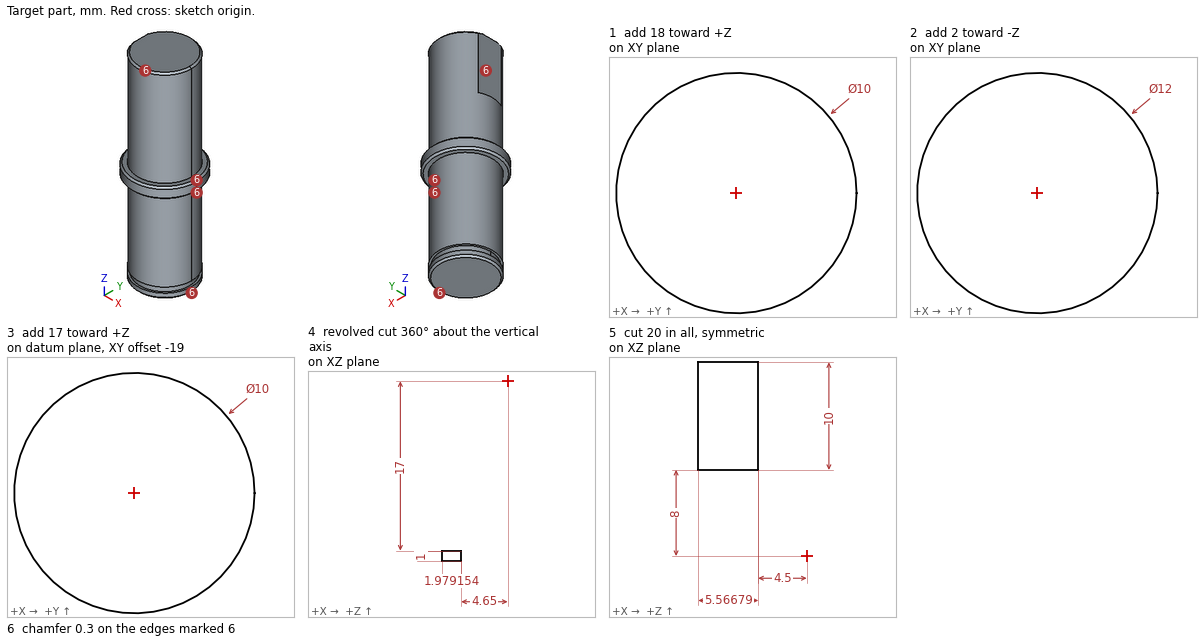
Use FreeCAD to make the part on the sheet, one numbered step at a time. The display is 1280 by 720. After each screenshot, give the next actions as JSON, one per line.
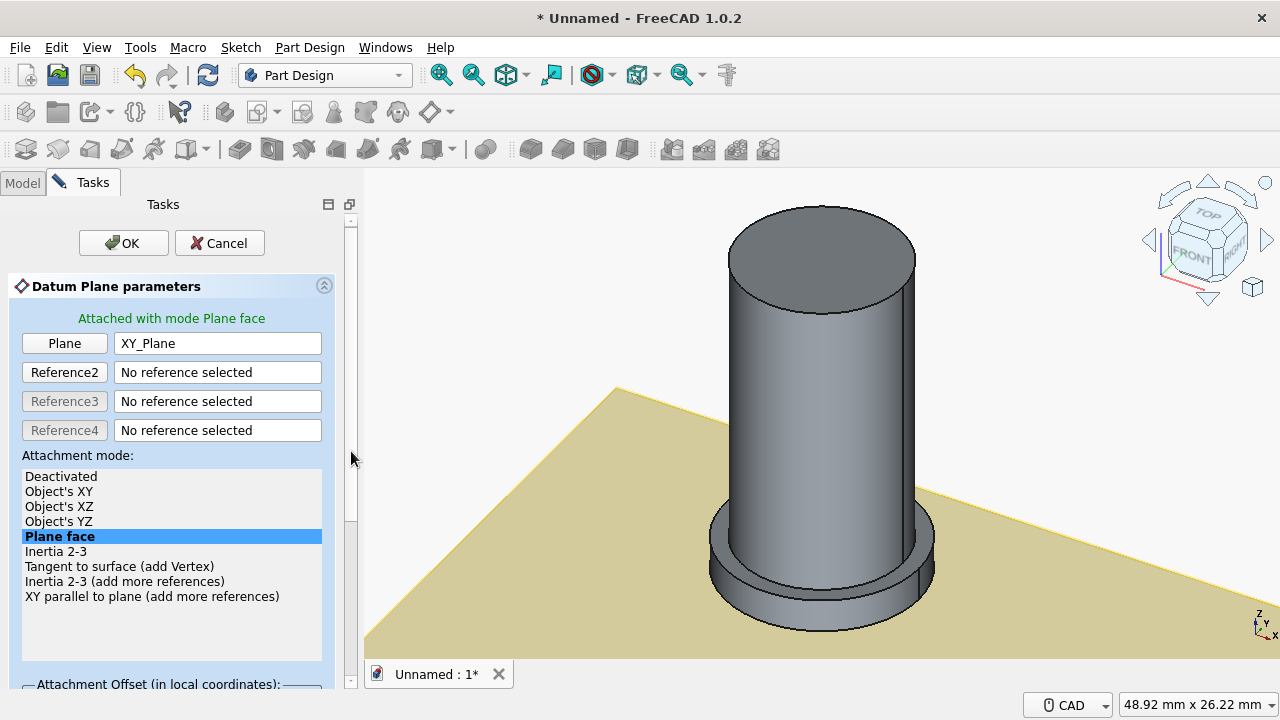
{"action": "left_click", "coordinate": [124, 243]}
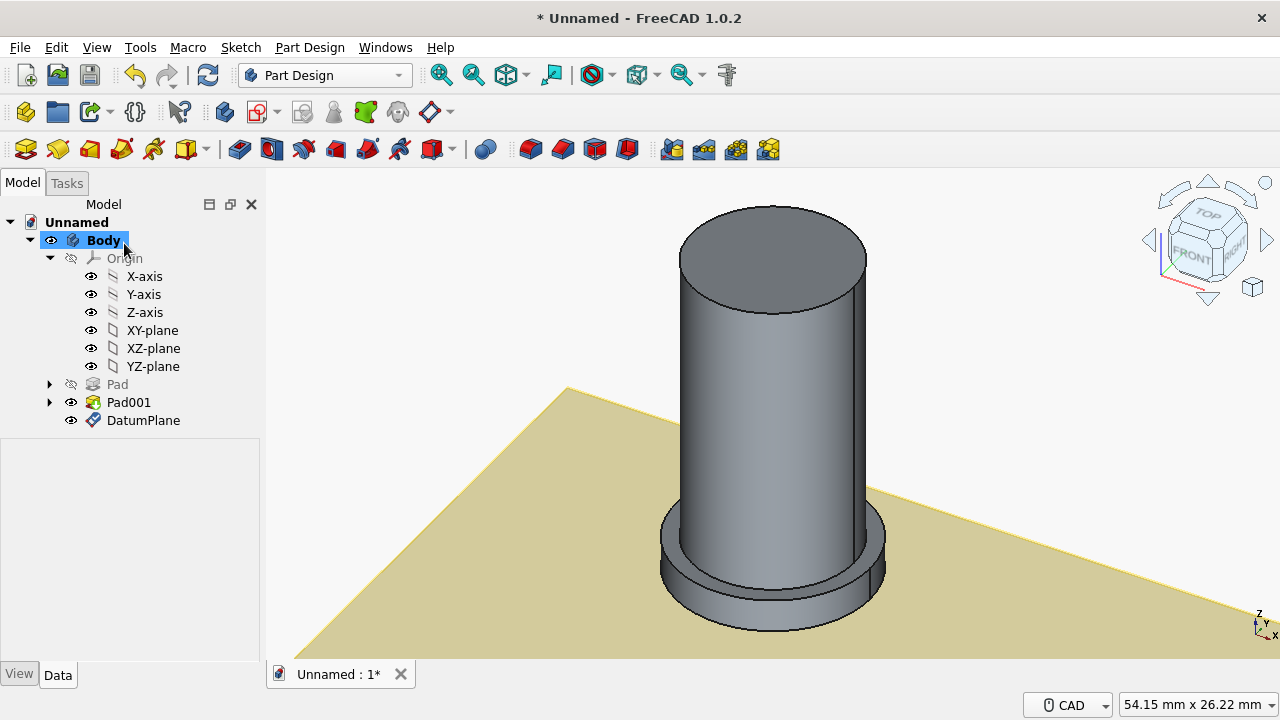
{"action": "left_click", "coordinate": [116, 420]}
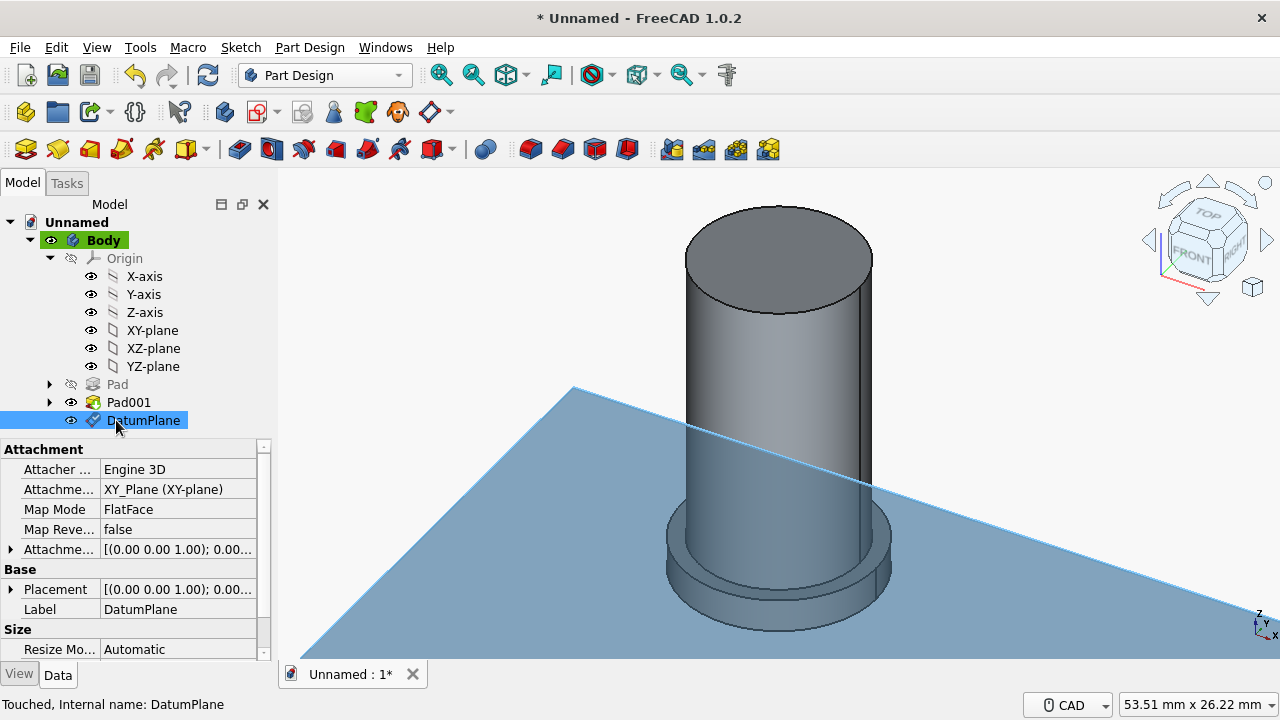
{"action": "left_click", "coordinate": [258, 112]}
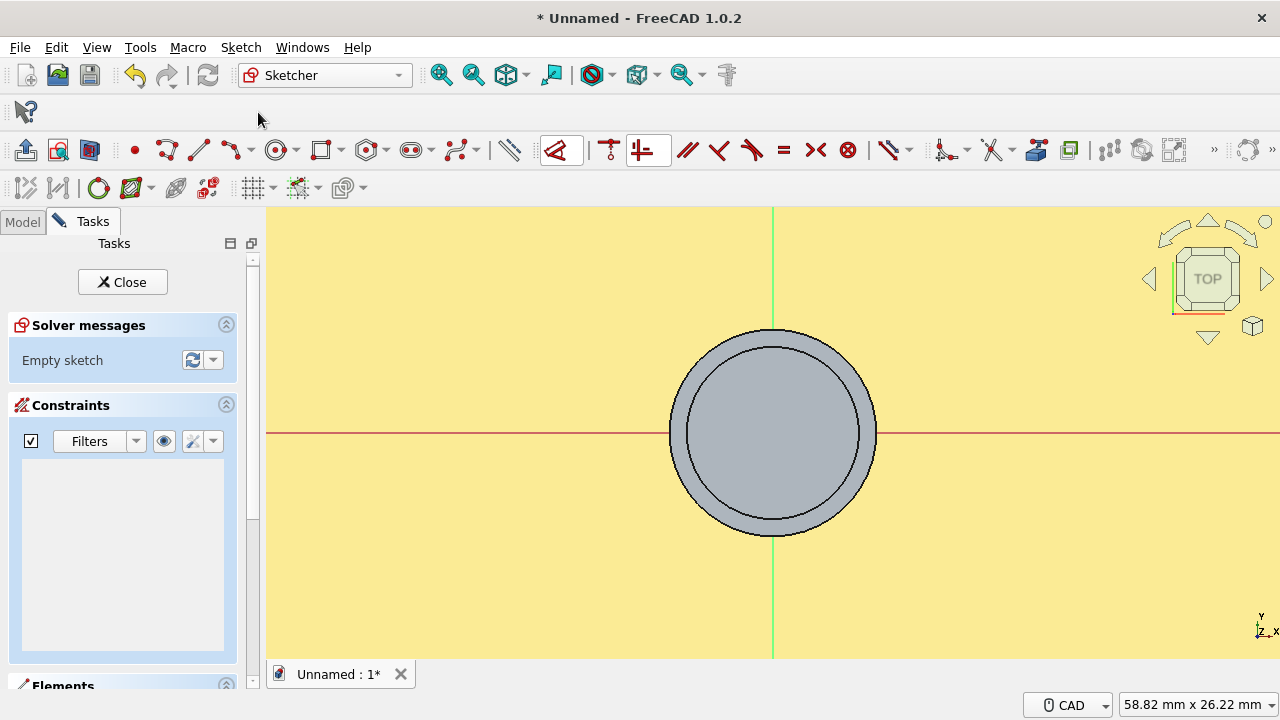
{"action": "left_click", "coordinate": [90, 150]}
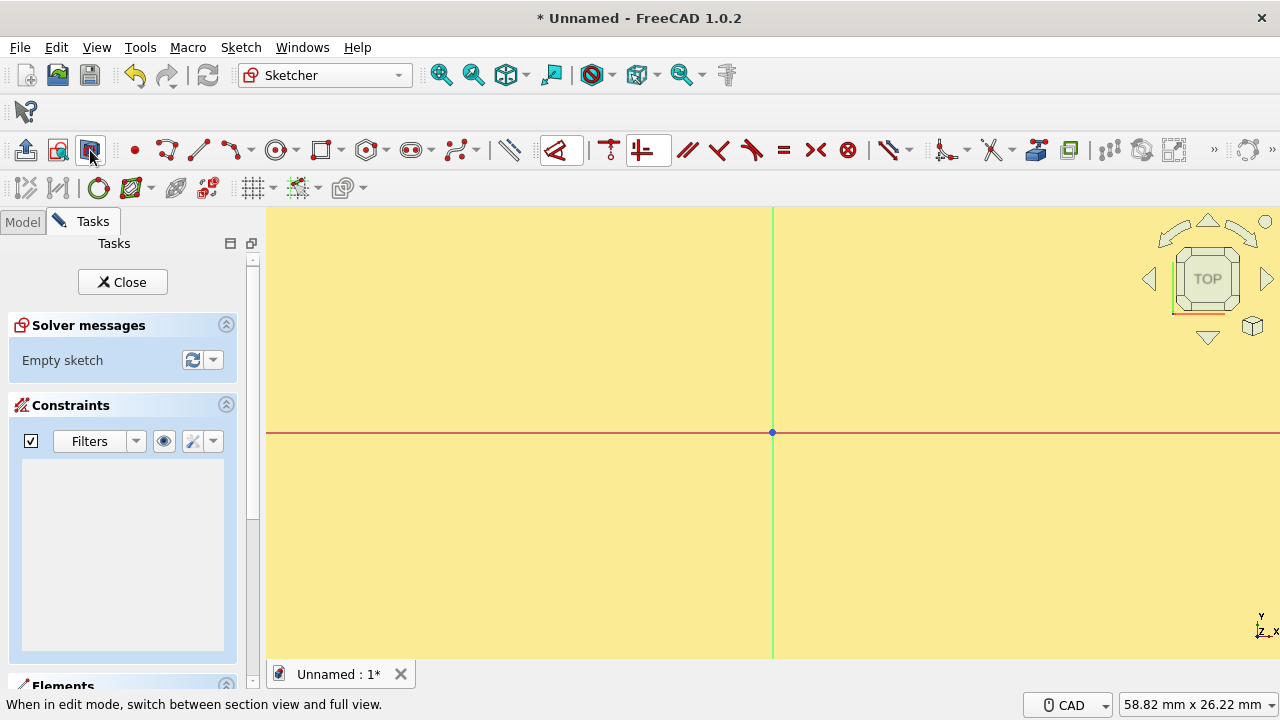
{"action": "scroll", "coordinate": [912, 433], "scroll_direction": "up", "scroll_amount": 2}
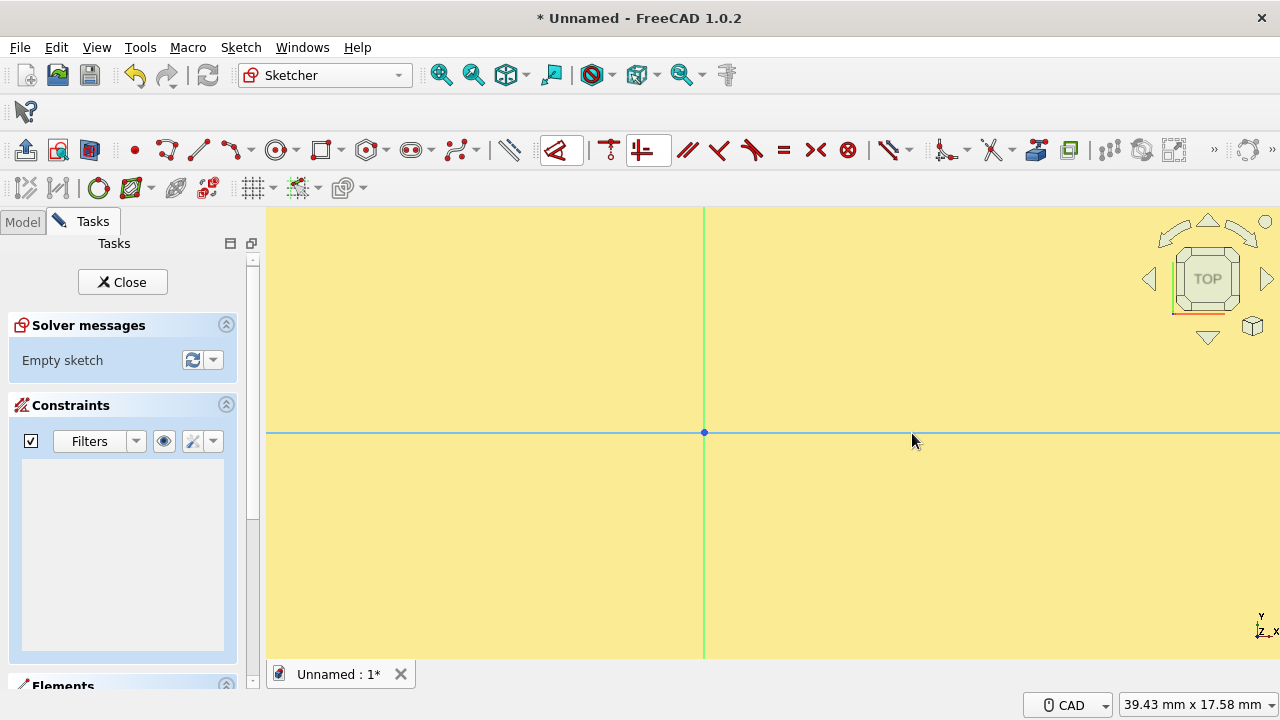
{"action": "left_click", "coordinate": [276, 150]}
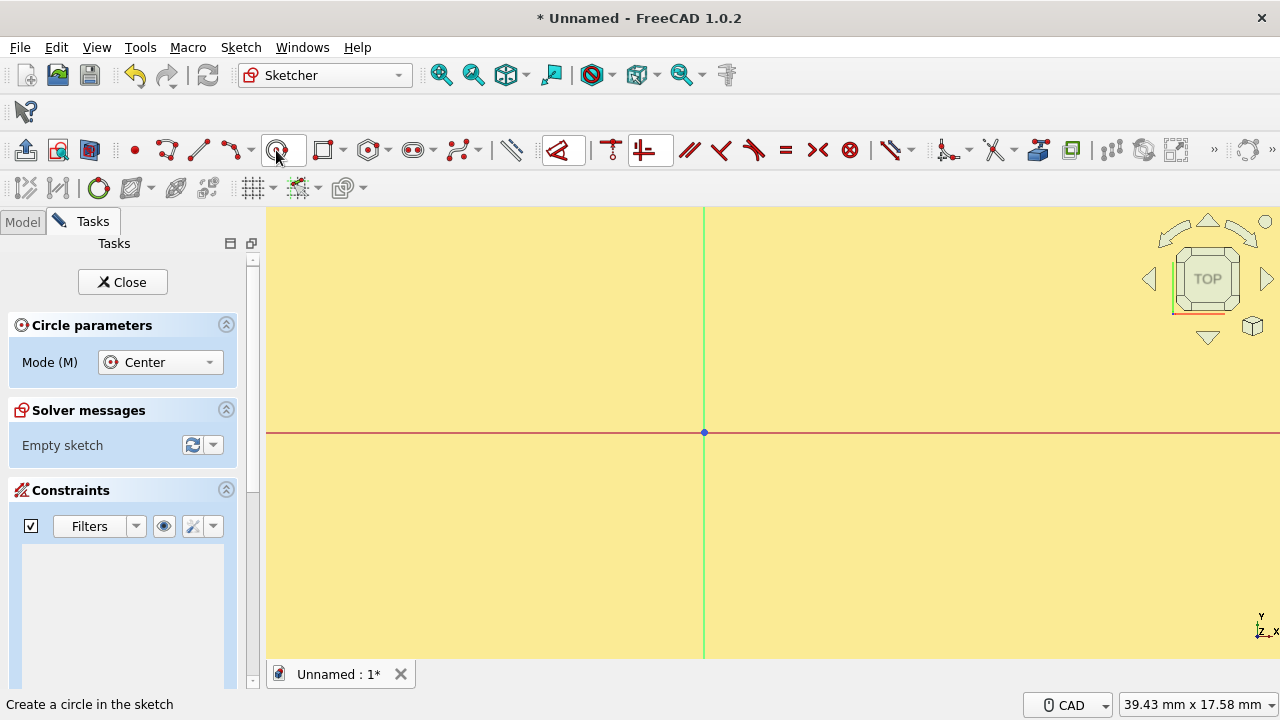
{"action": "left_click", "coordinate": [704, 433]}
{"action": "mouse_move", "coordinate": [795, 342]}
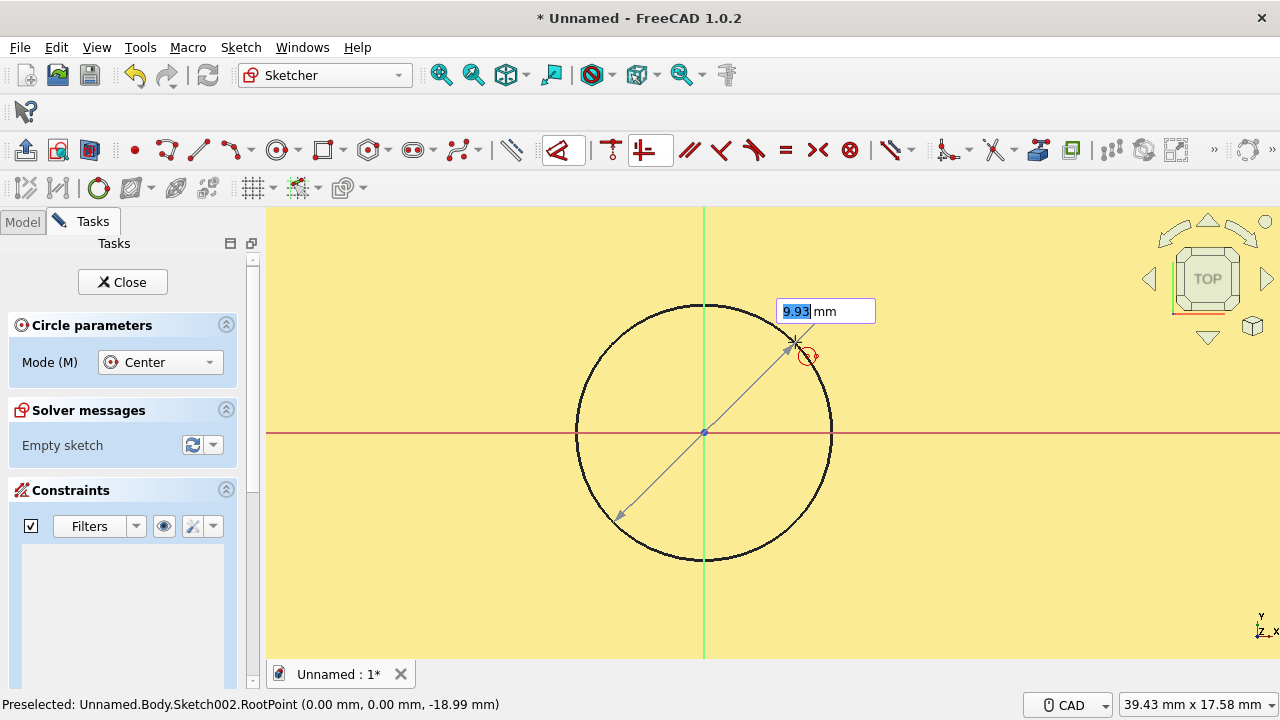
{"action": "type", "text": "10"}
{"action": "key", "text": "Return"}
{"action": "key", "text": "Escape"}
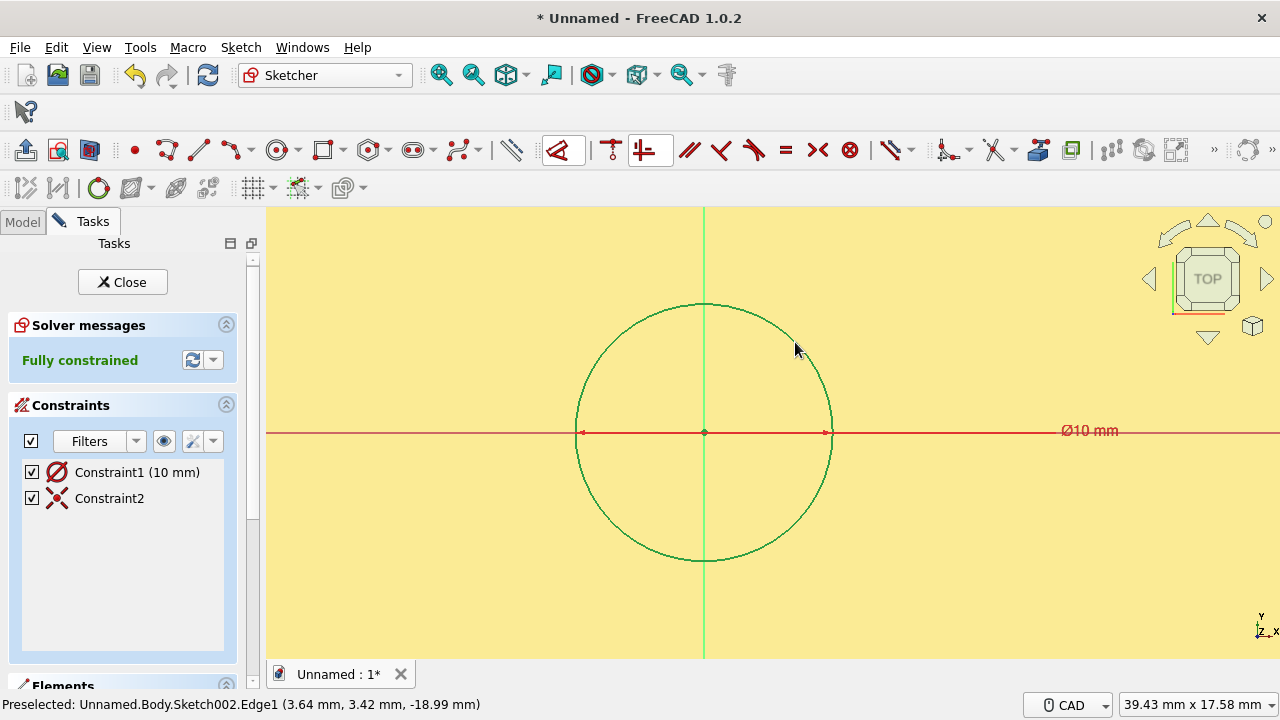
{"action": "left_click", "coordinate": [123, 282]}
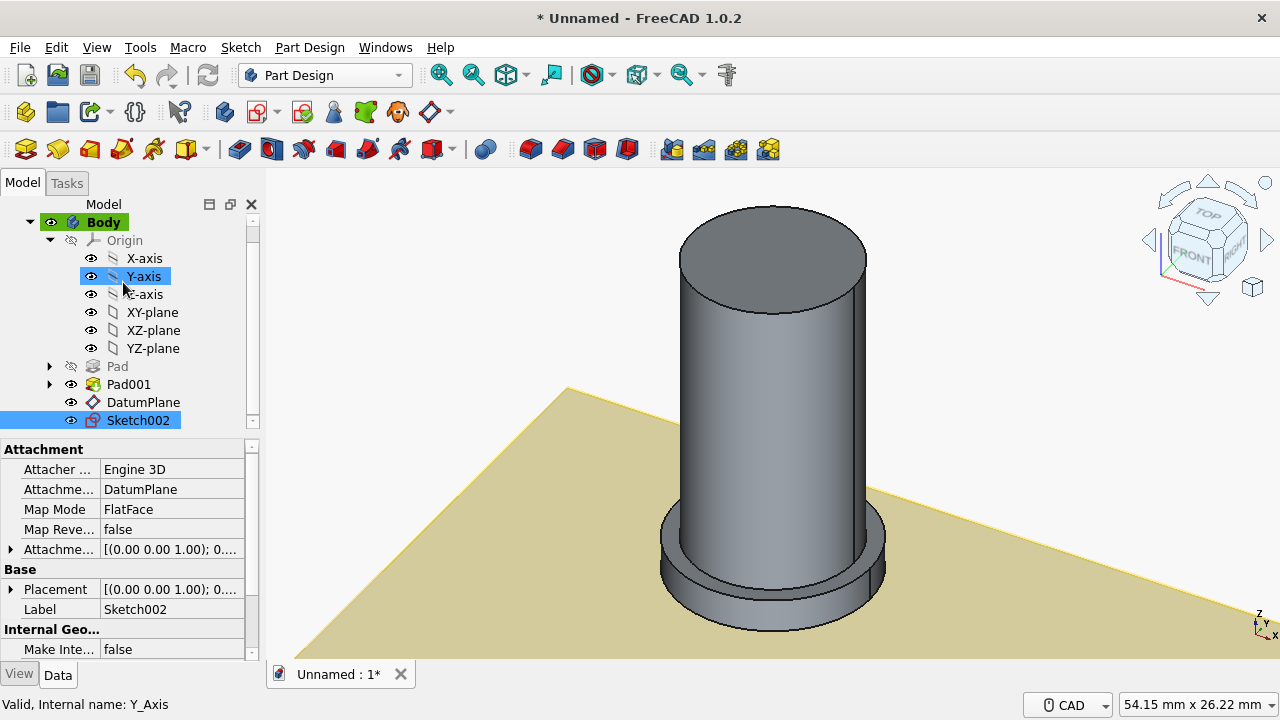
{"action": "left_click", "coordinate": [26, 150]}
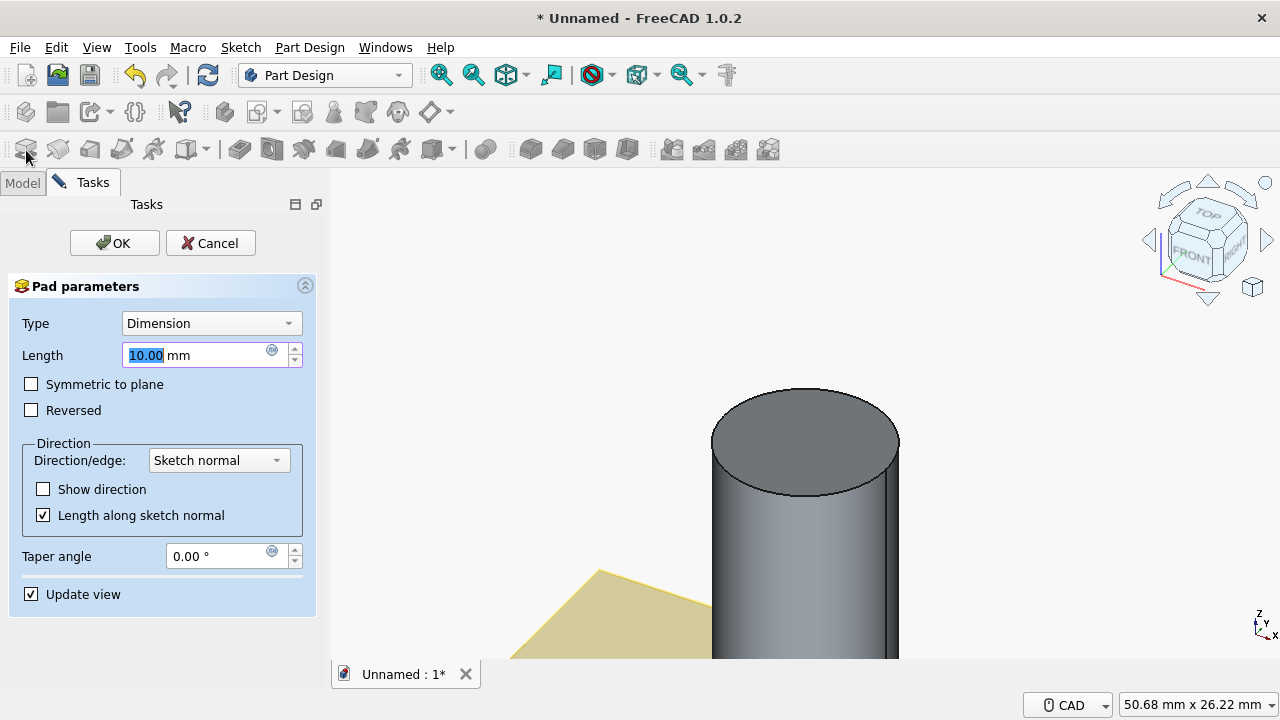
{"action": "type", "text": "17"}
{"action": "key", "text": "Tab"}